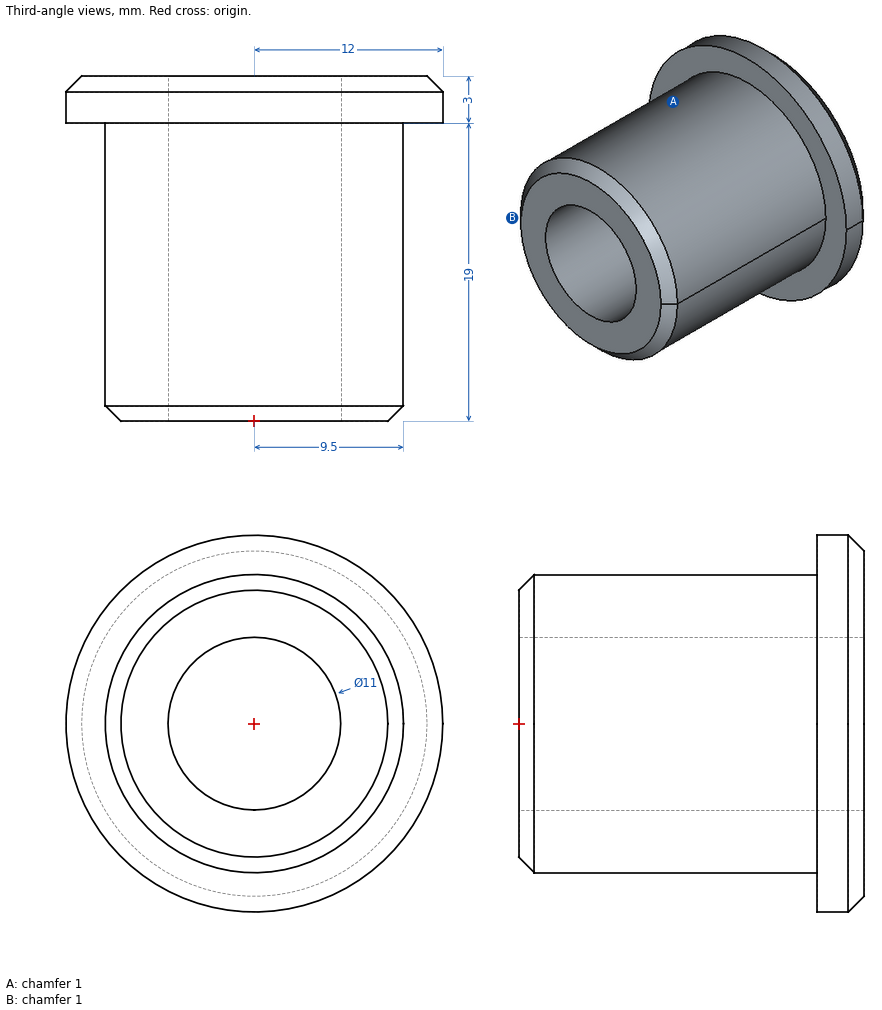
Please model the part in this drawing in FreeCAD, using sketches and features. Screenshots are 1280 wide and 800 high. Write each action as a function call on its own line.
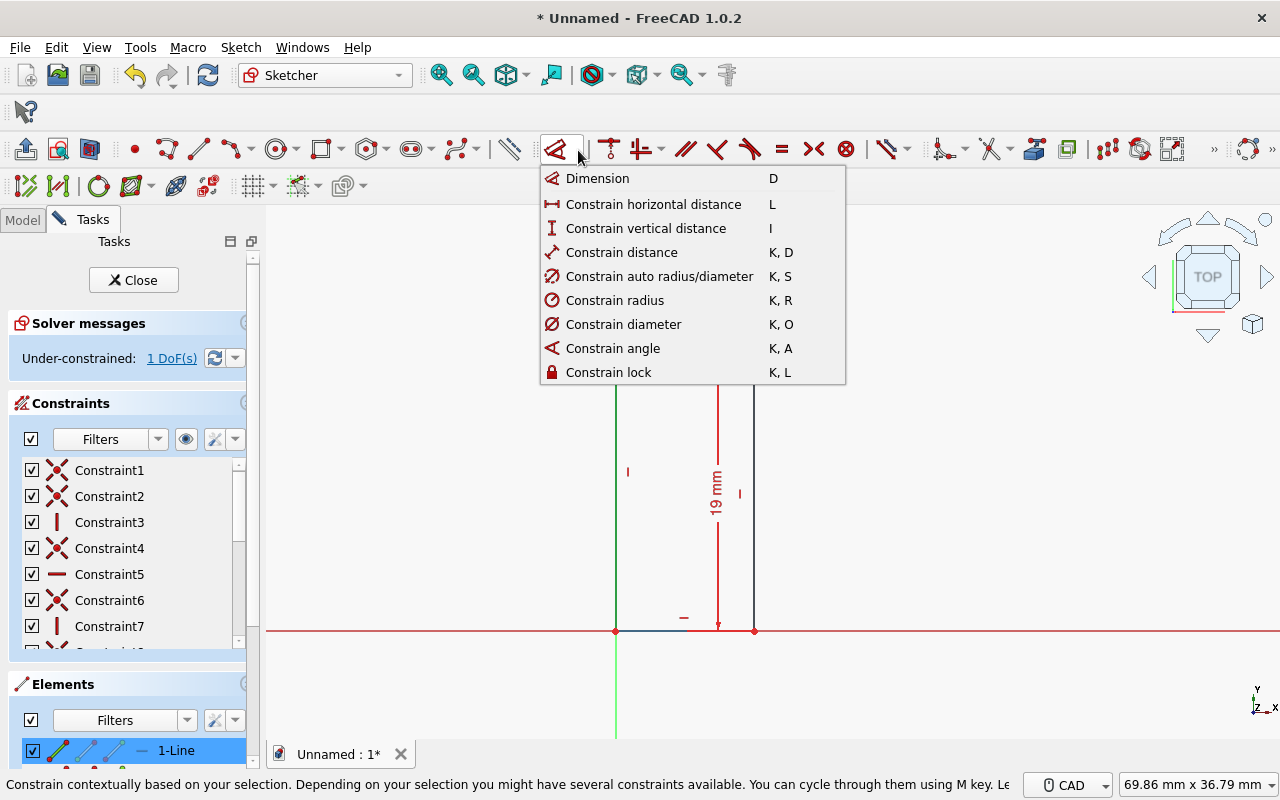
click(693, 204)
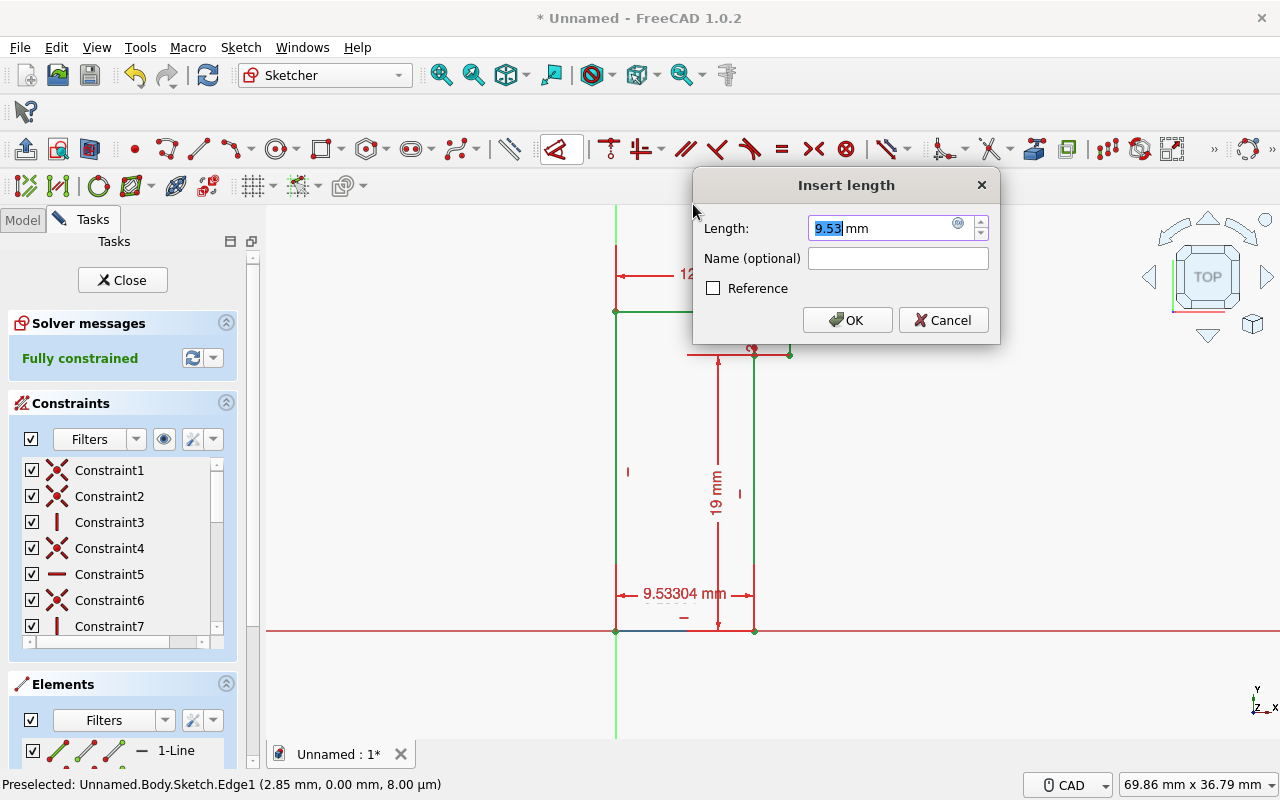
text(9.5)
key(Return)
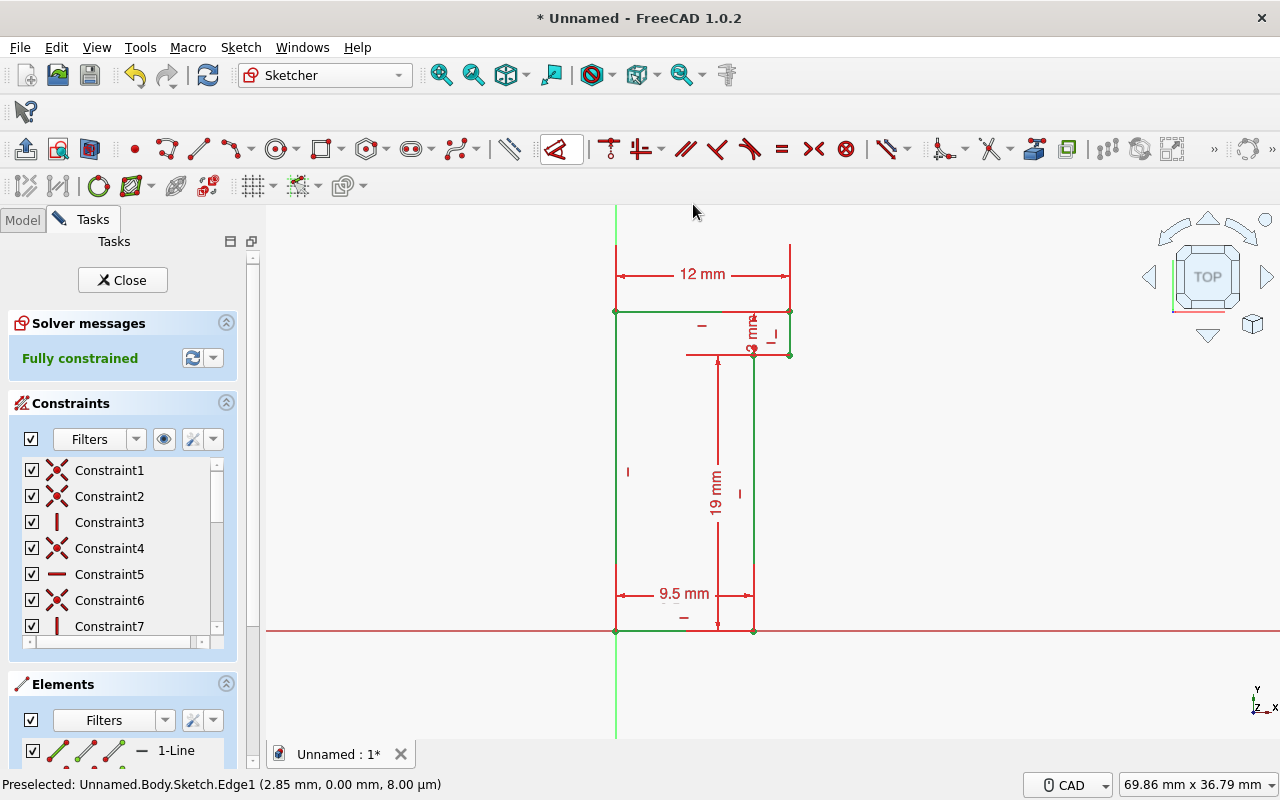
click(123, 280)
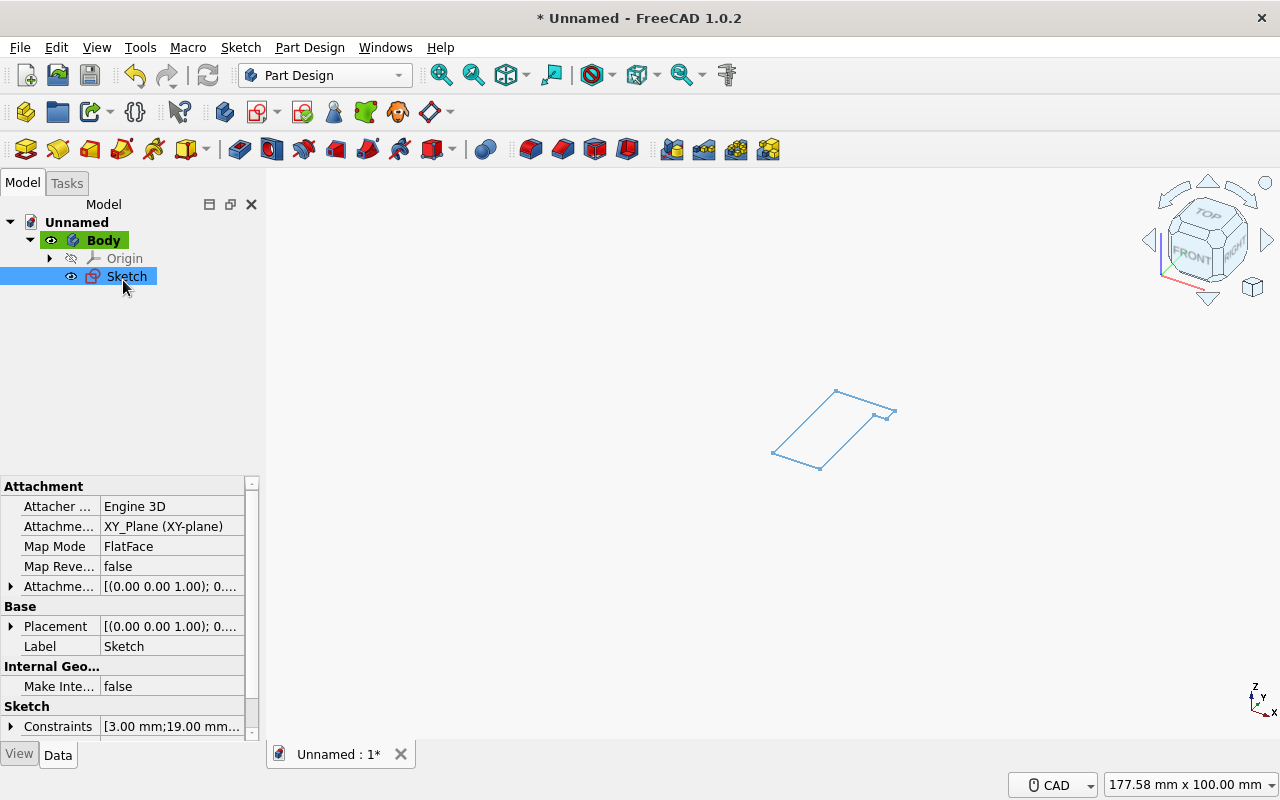
click(58, 150)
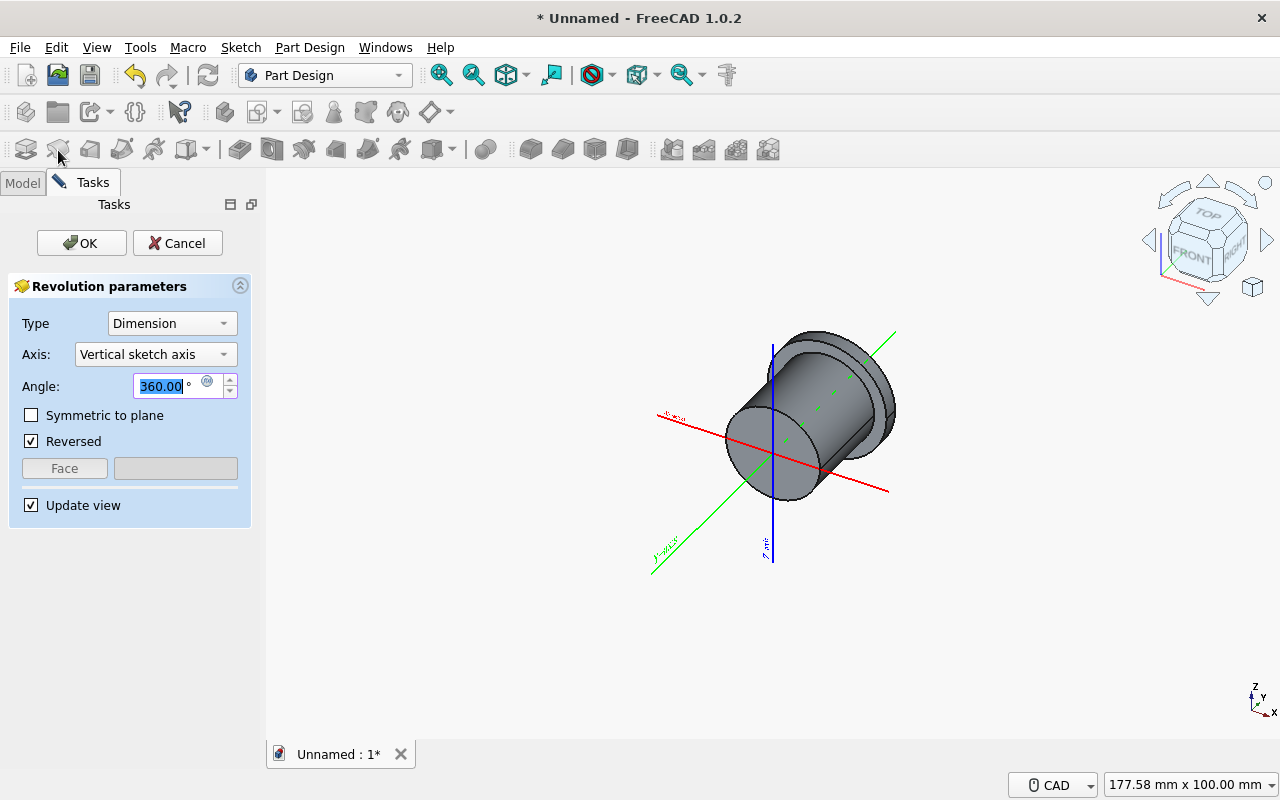
click(82, 243)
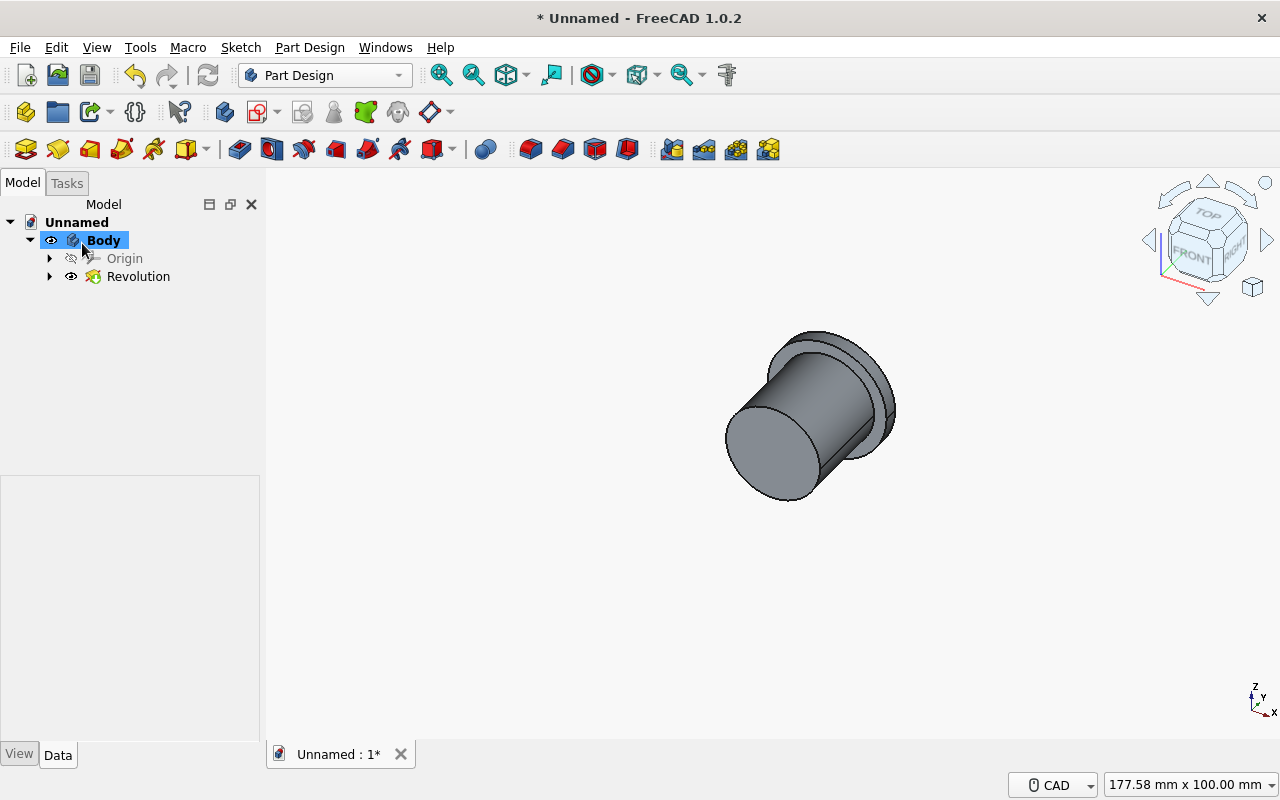
click(442, 76)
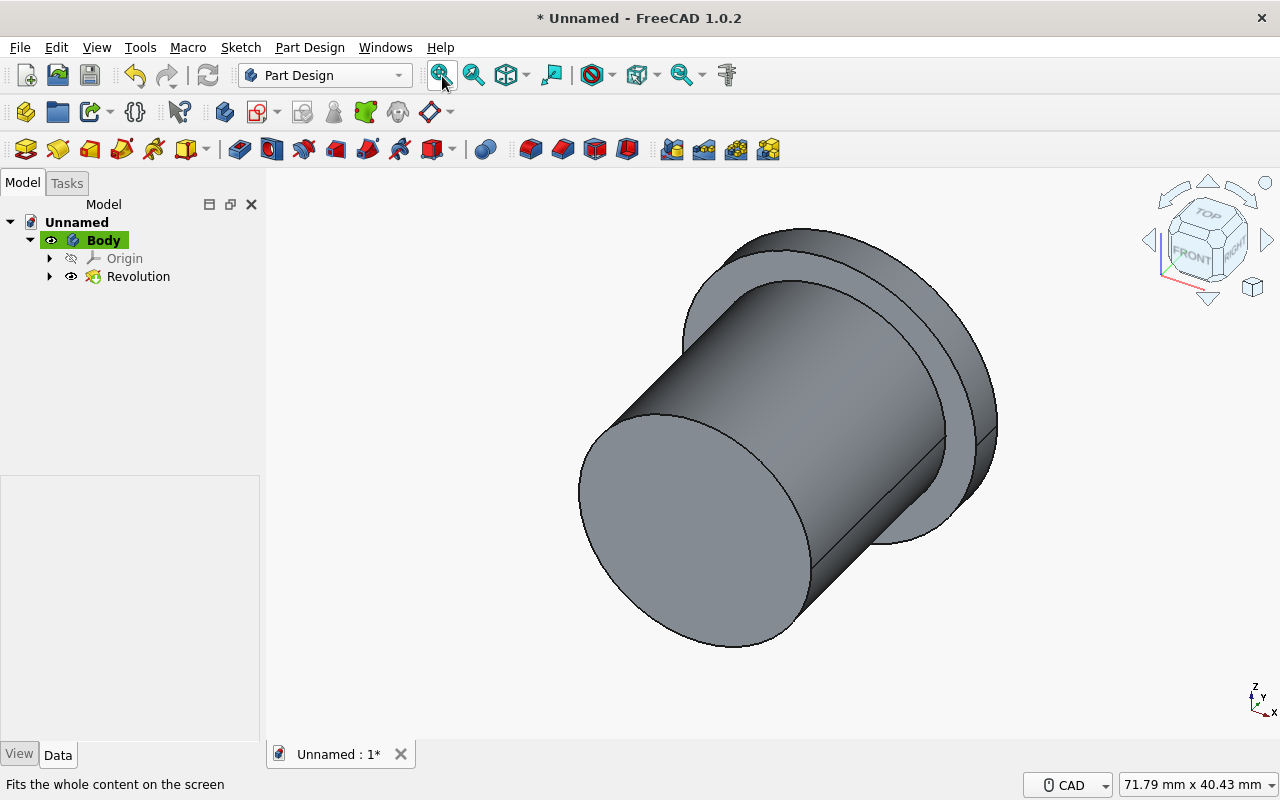
click(258, 112)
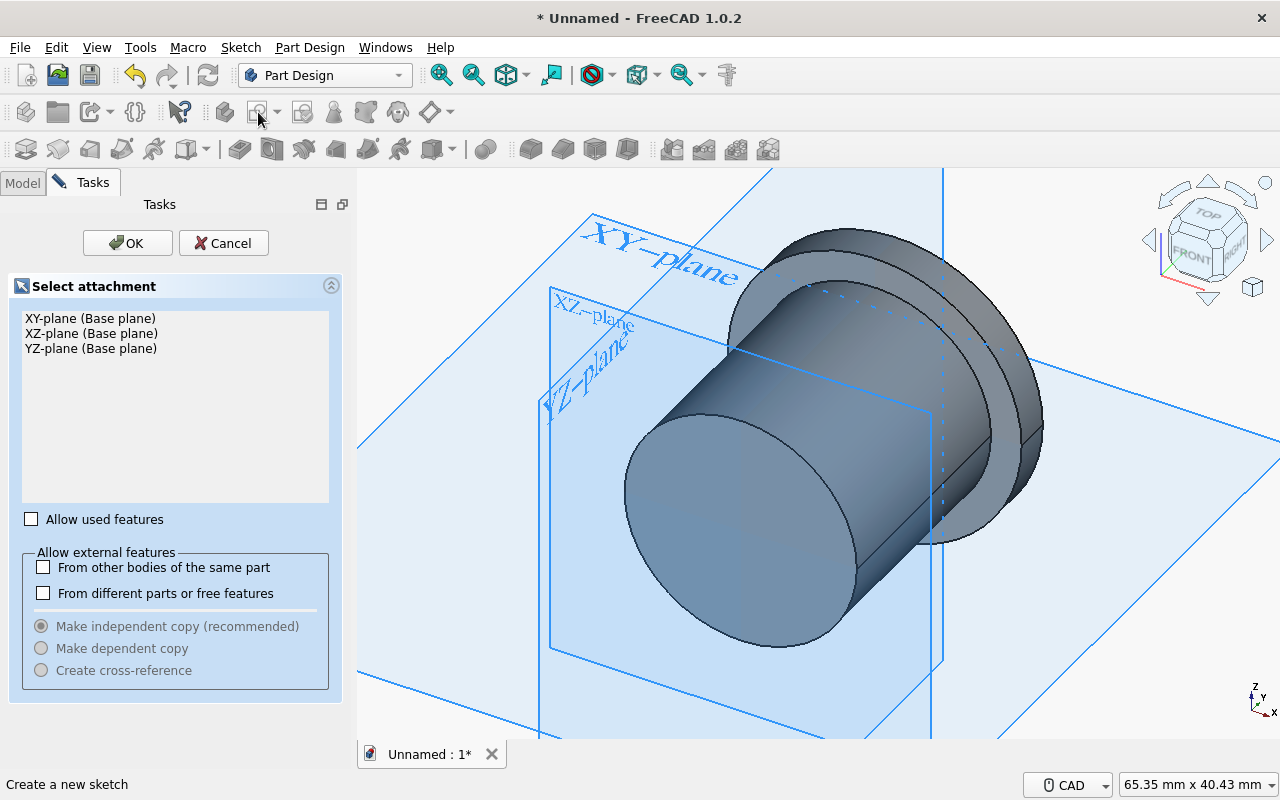
click(82, 334)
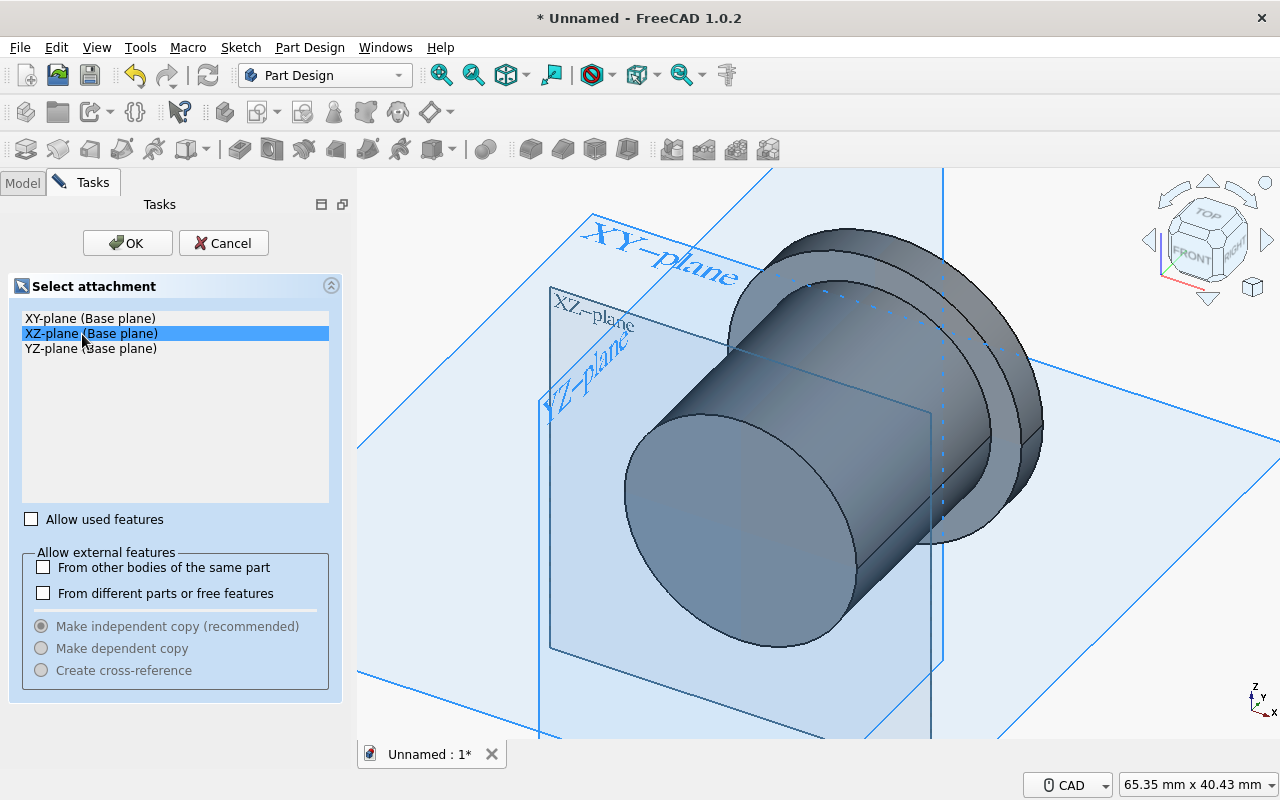
click(128, 243)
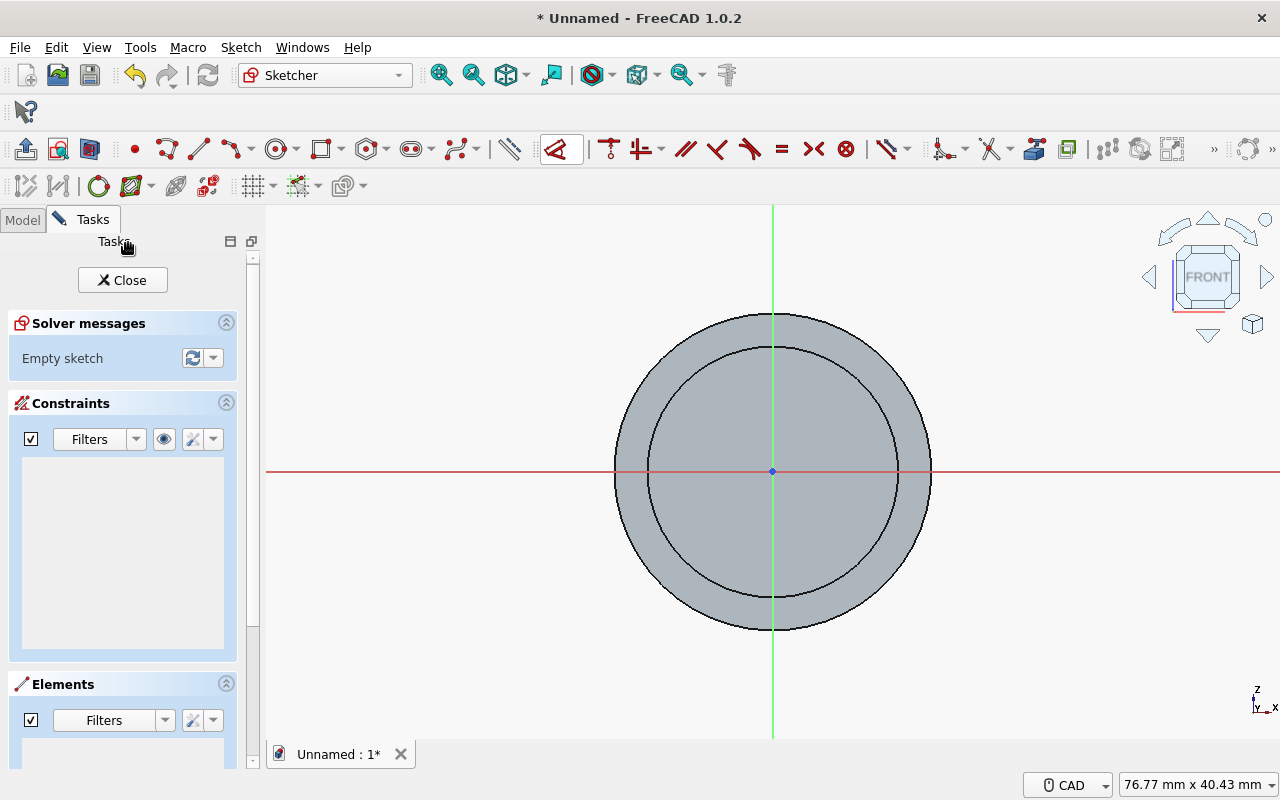
scroll(829, 472, up, 4)